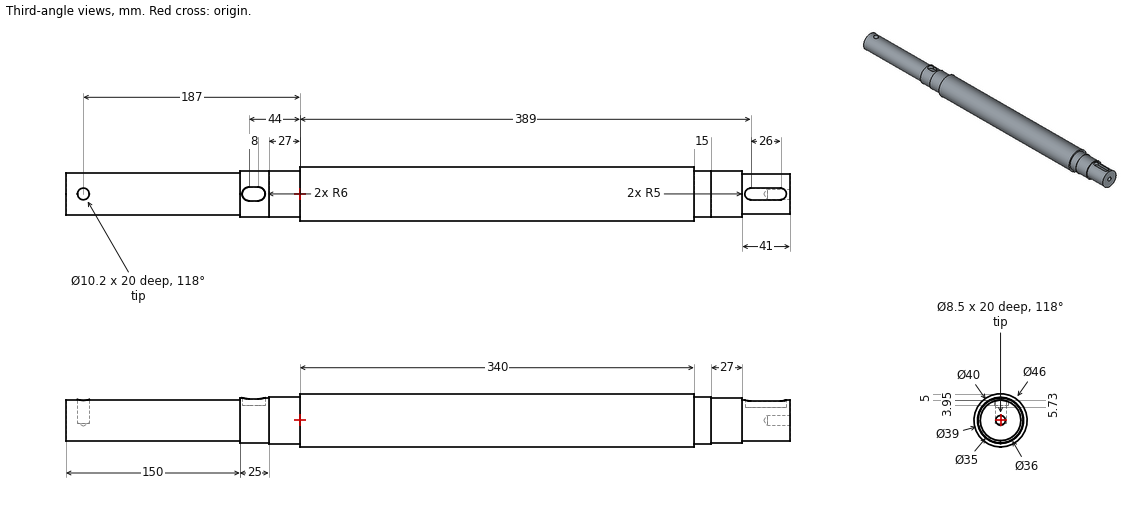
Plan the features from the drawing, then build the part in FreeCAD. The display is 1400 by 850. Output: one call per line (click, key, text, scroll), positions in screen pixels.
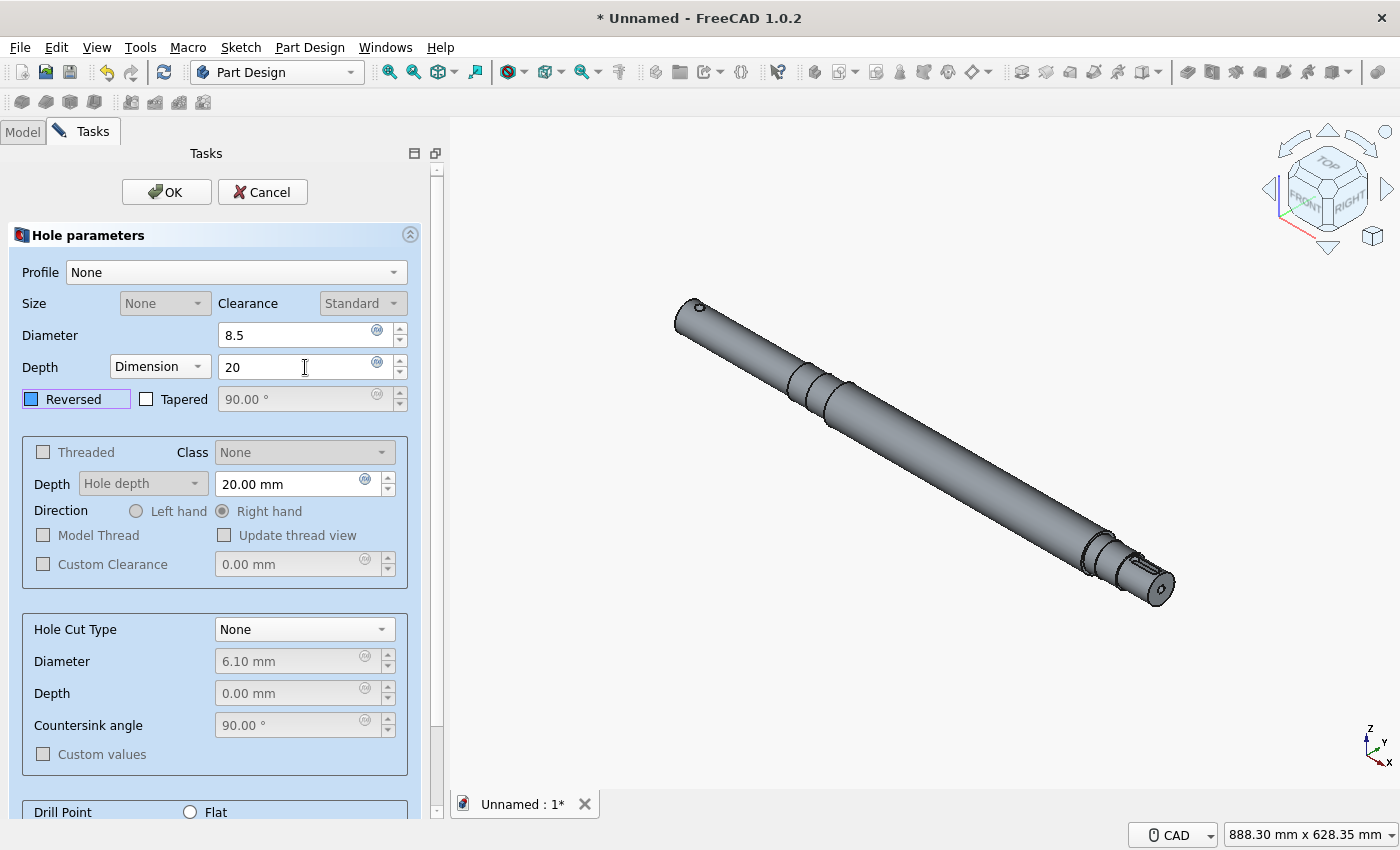
click(167, 192)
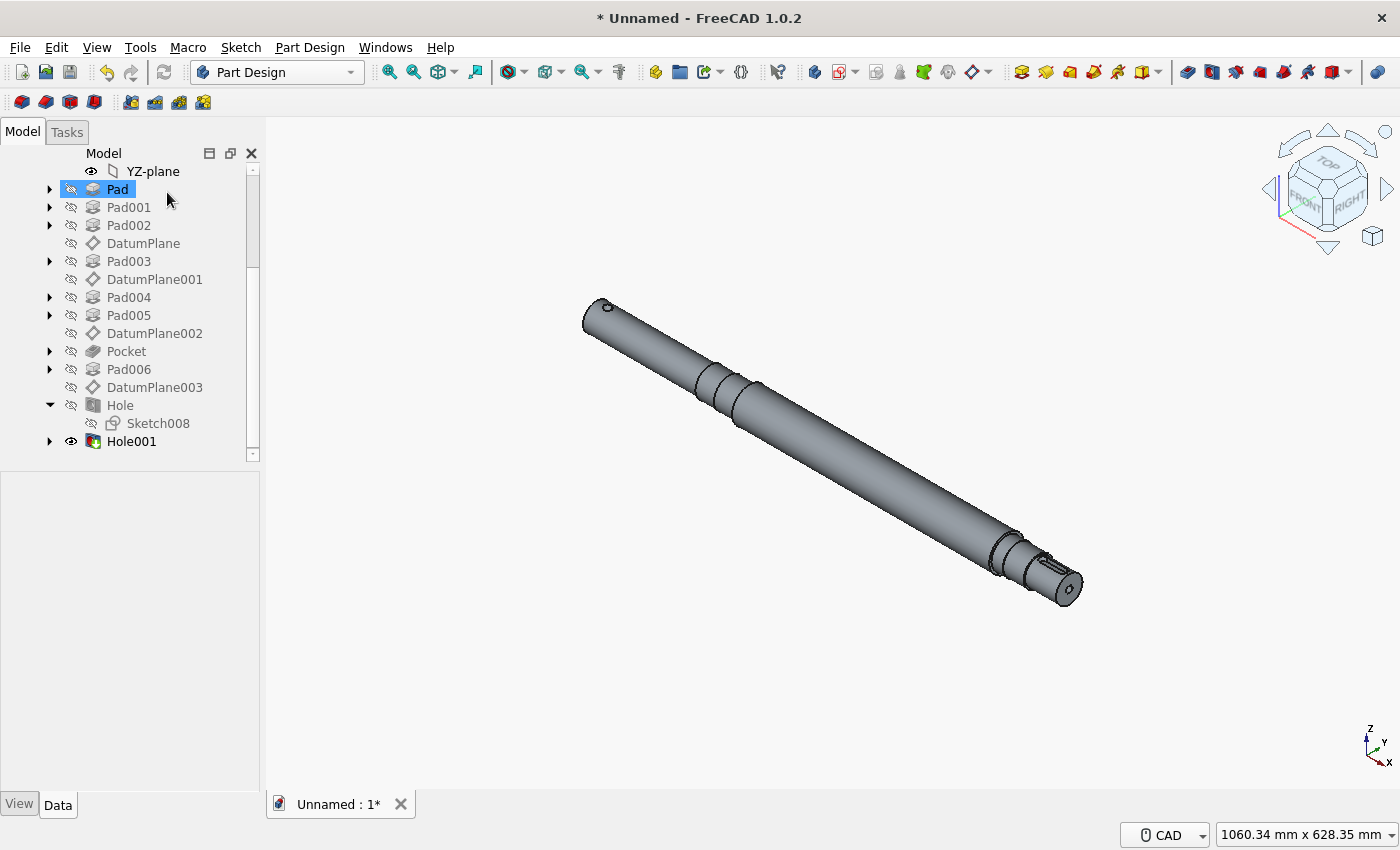
scroll(160, 311, down, 3)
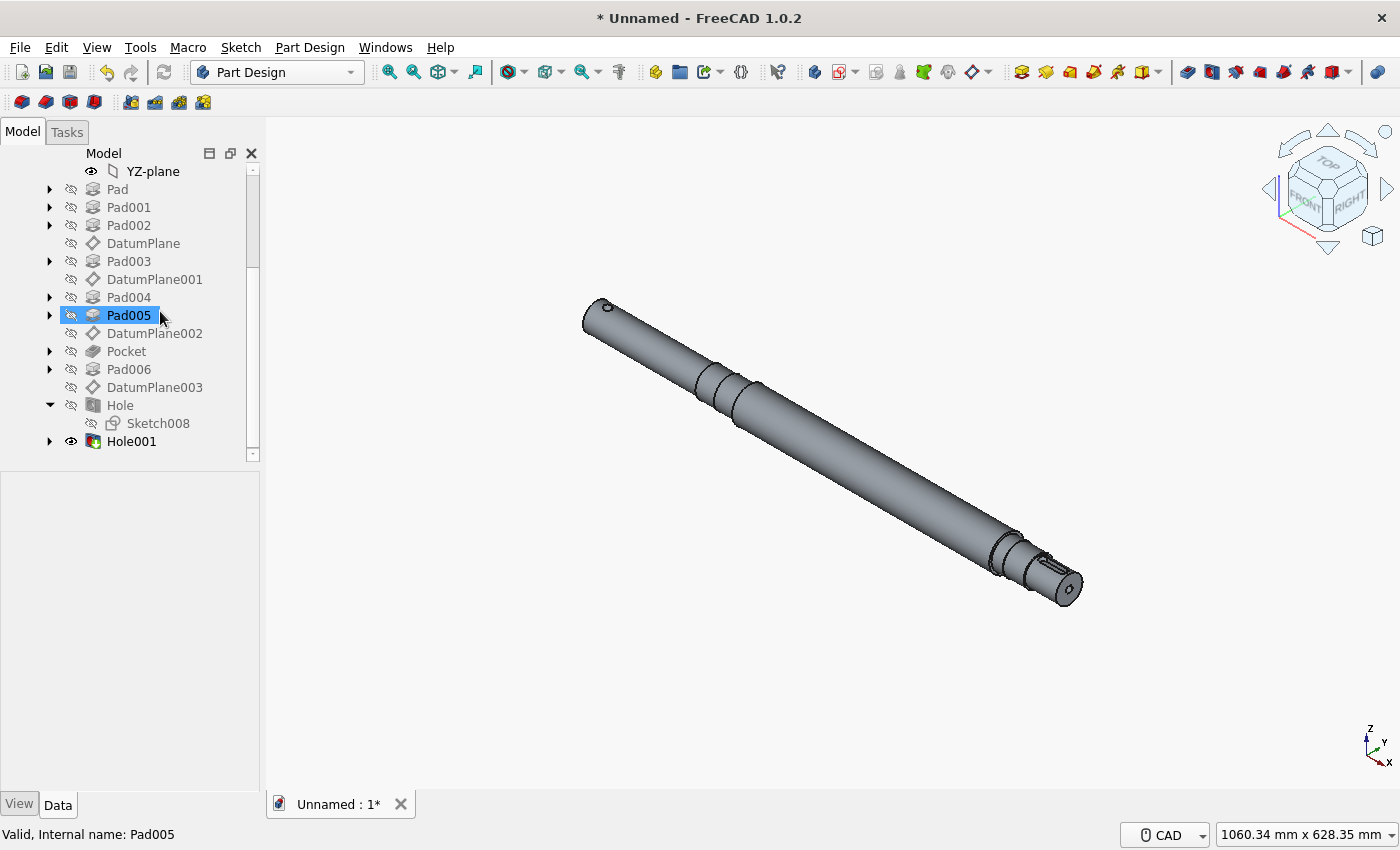
scroll(160, 311, up, 15)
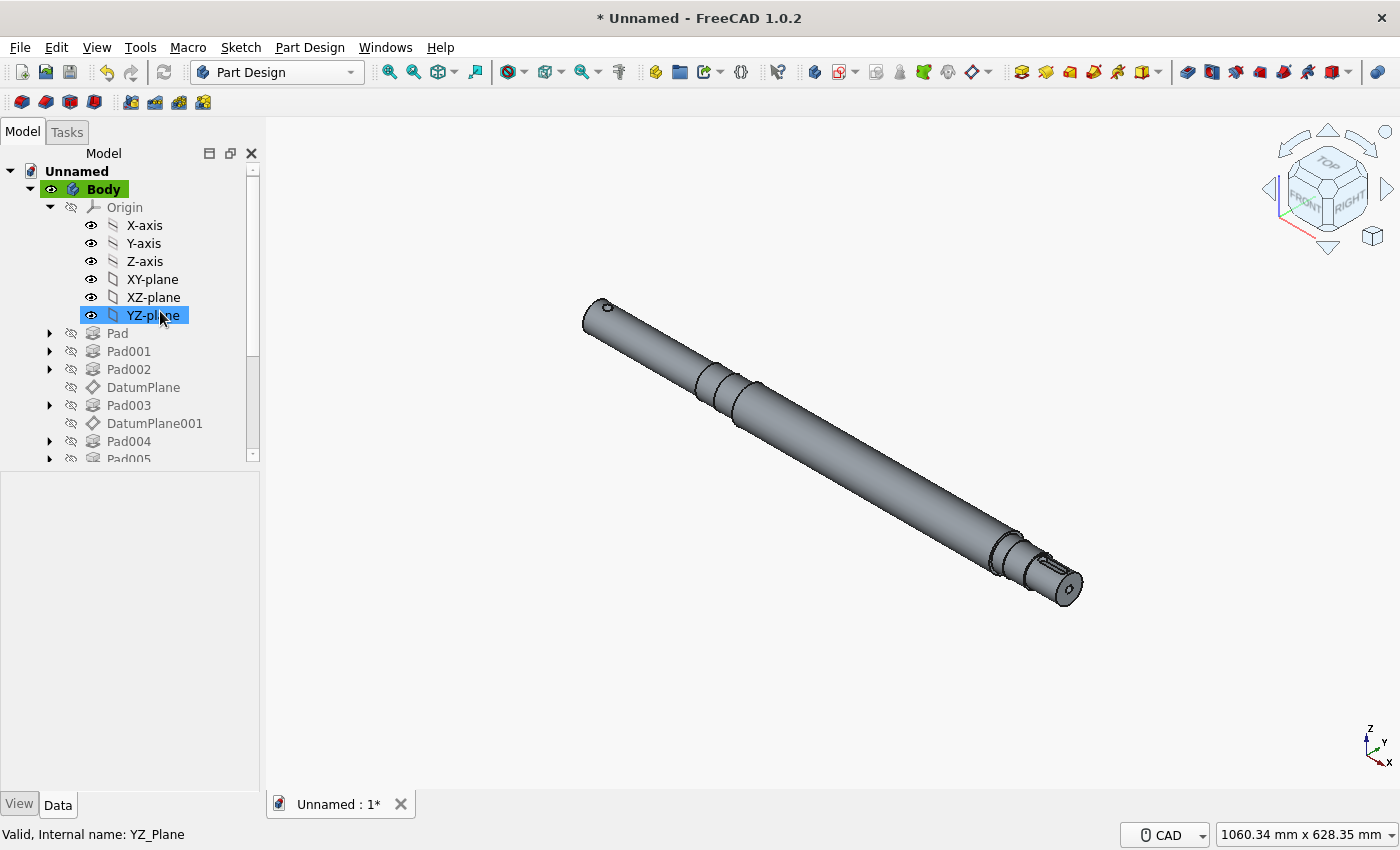
click(136, 279)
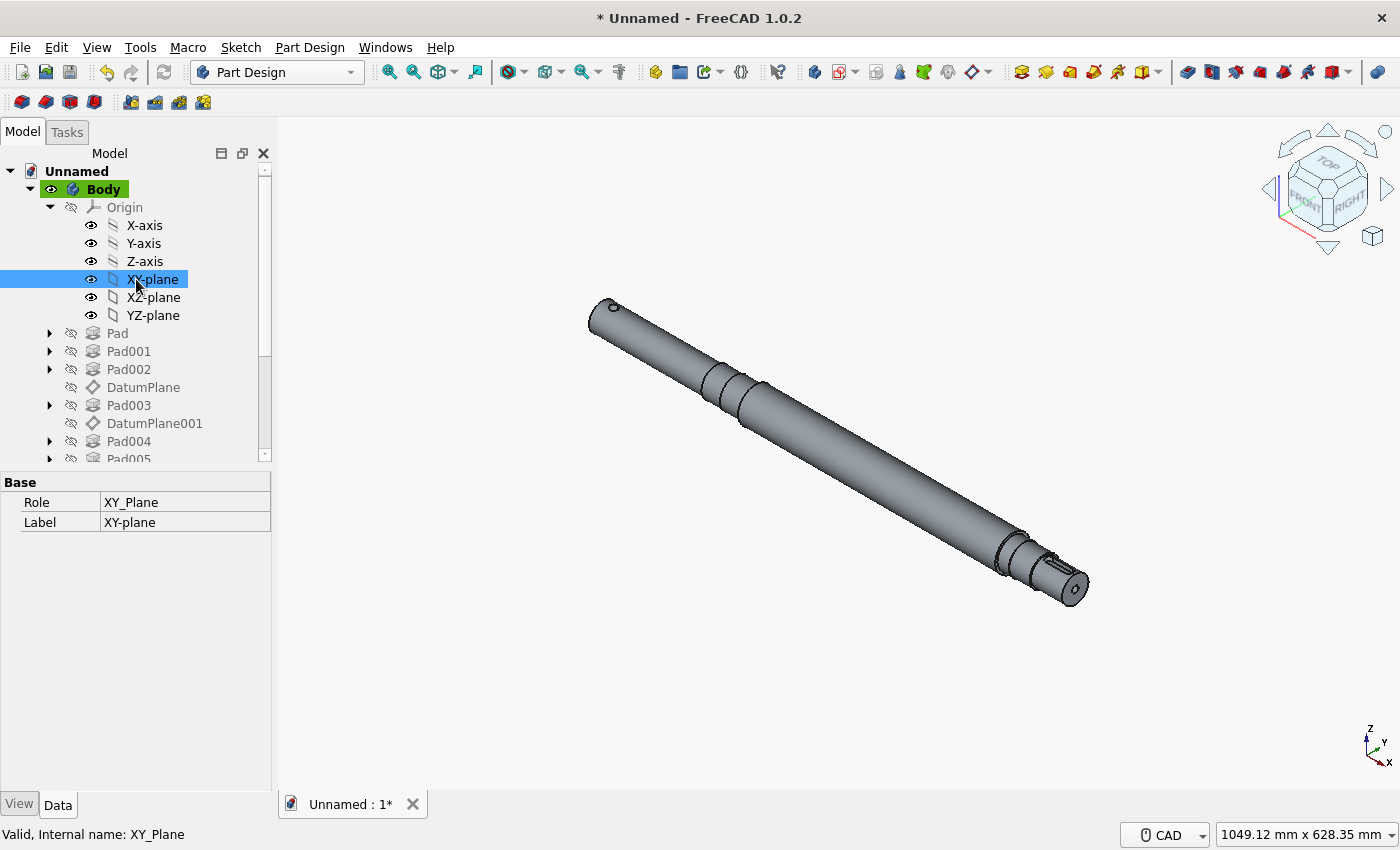
click(972, 72)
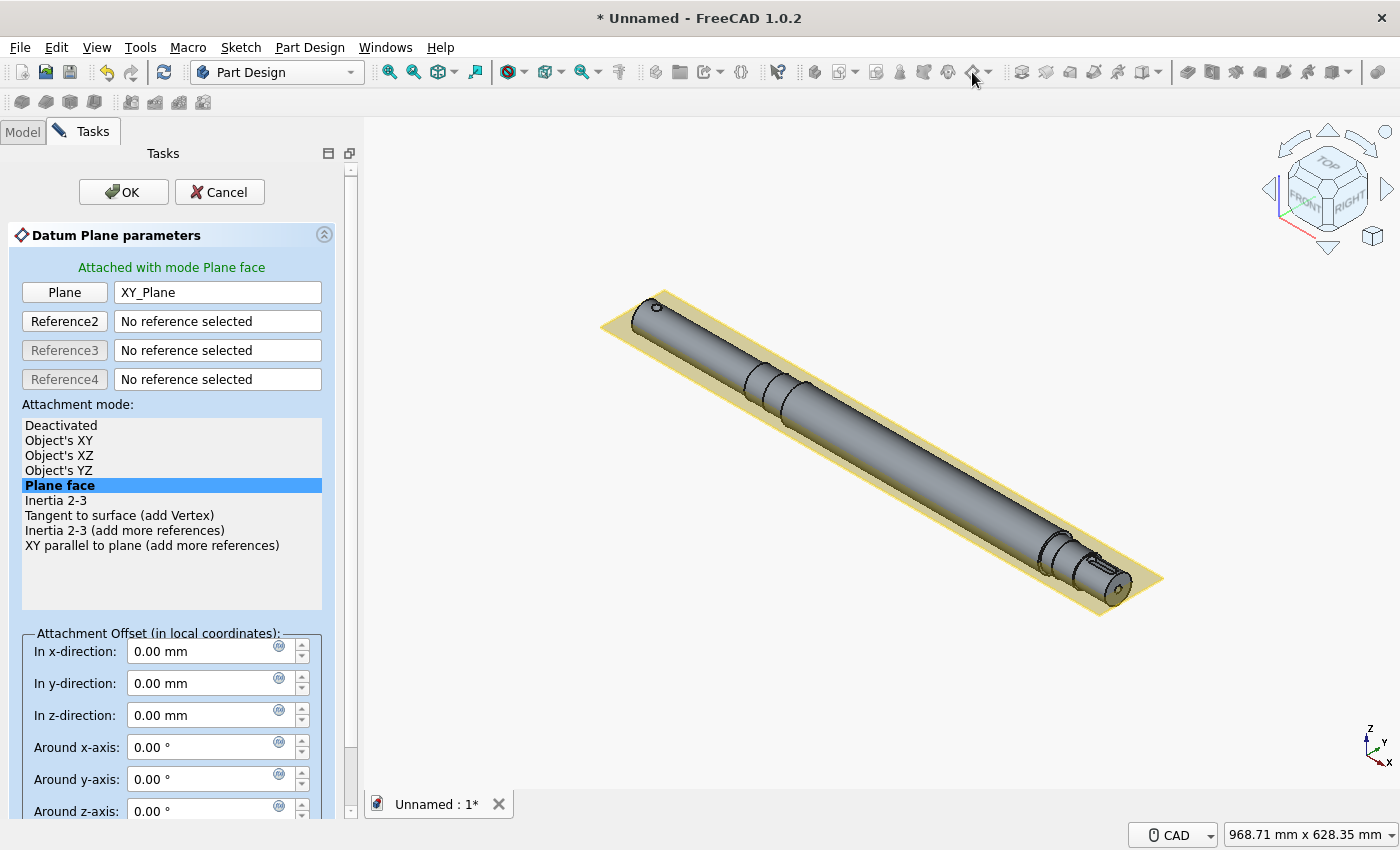
triple_click(210, 715)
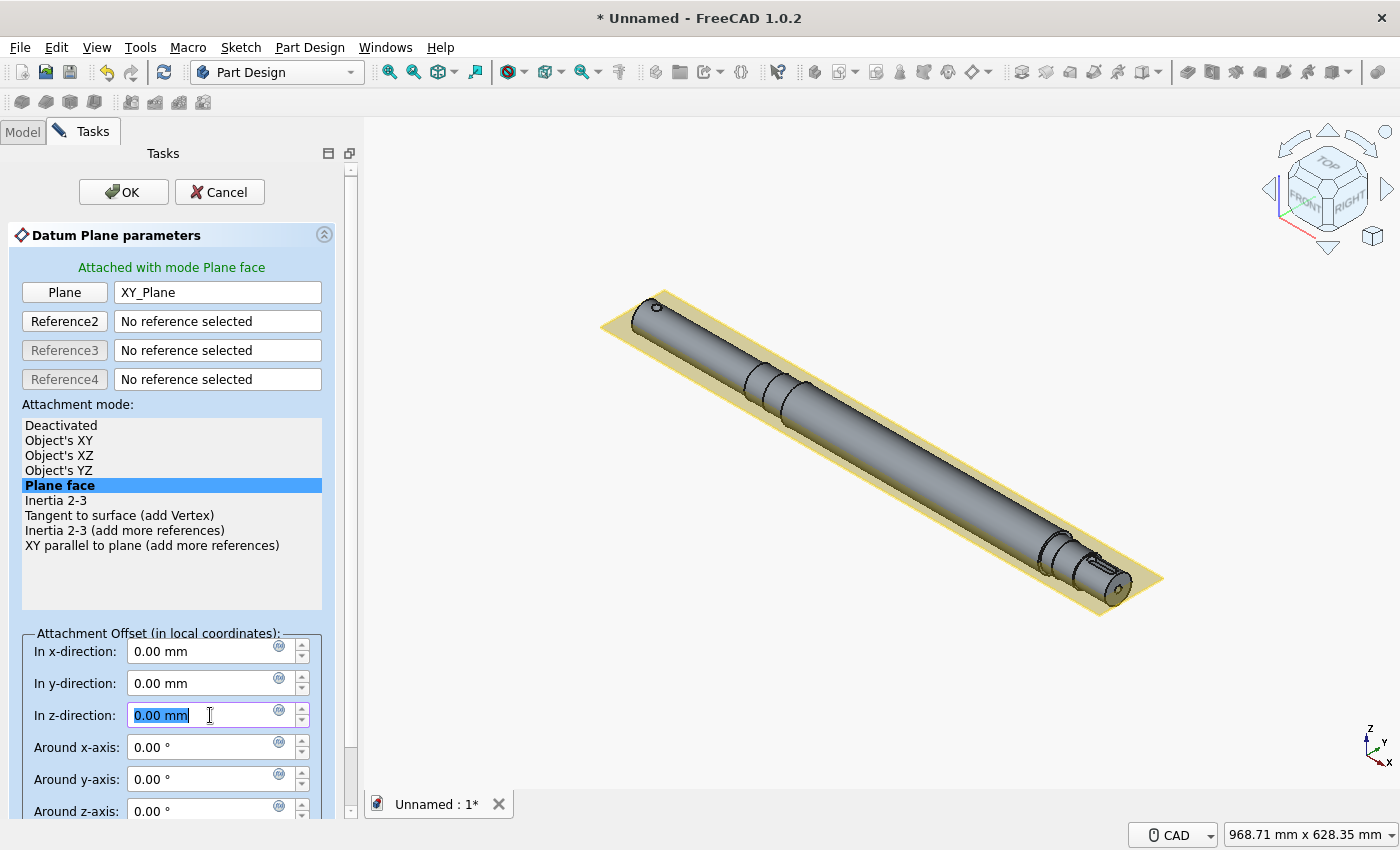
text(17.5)
key(Tab)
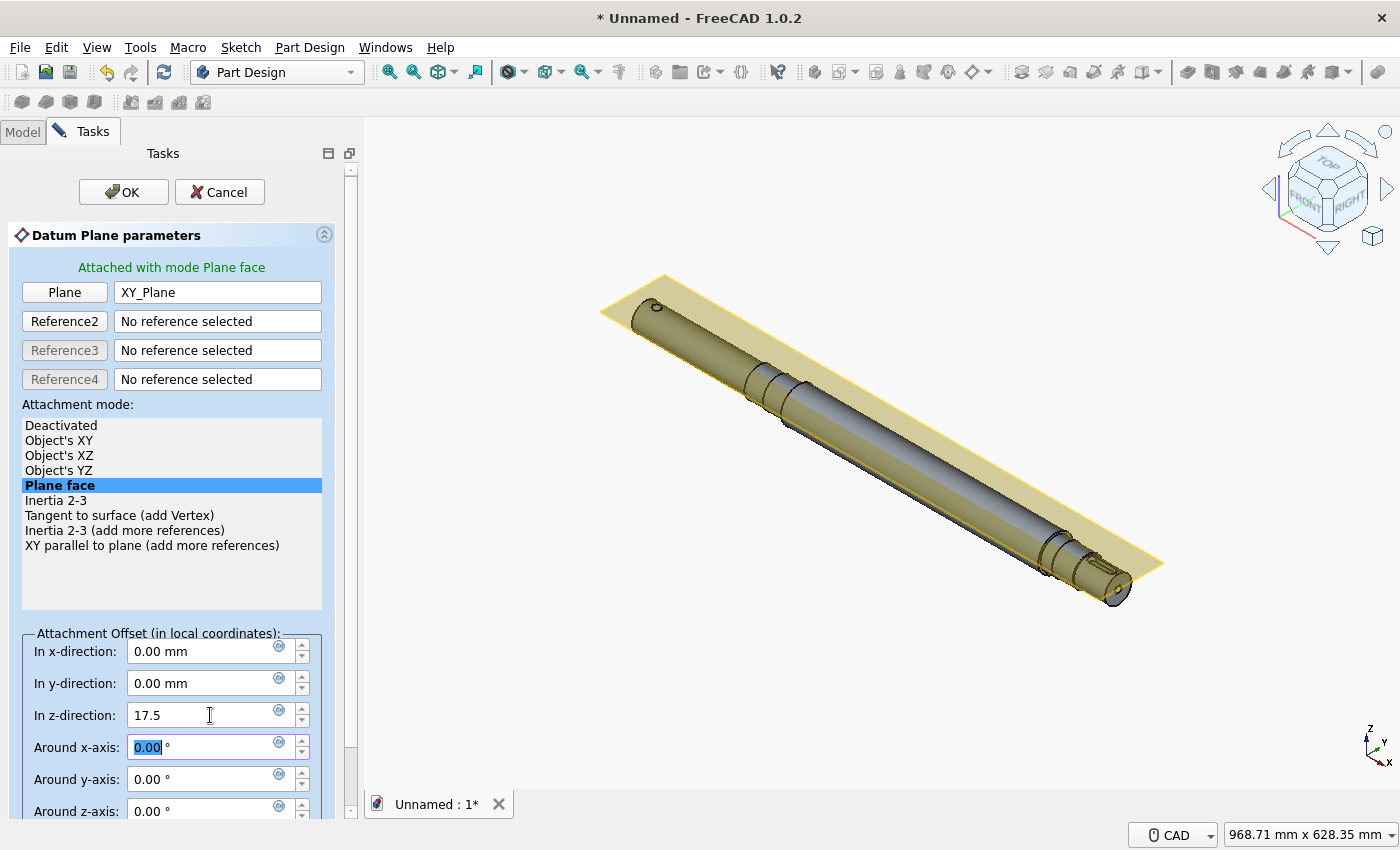
click(124, 192)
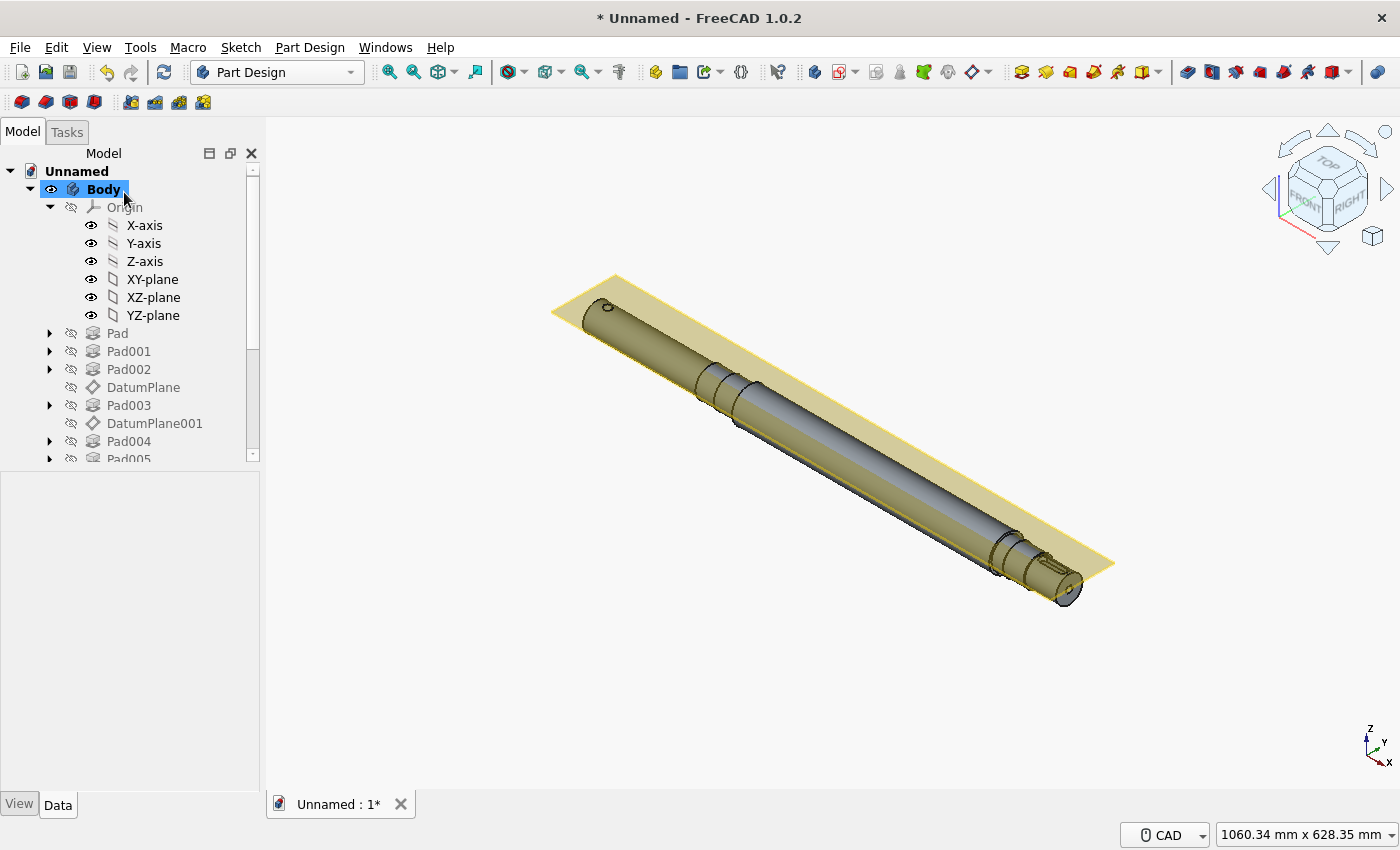
scroll(100, 311, down, 3)